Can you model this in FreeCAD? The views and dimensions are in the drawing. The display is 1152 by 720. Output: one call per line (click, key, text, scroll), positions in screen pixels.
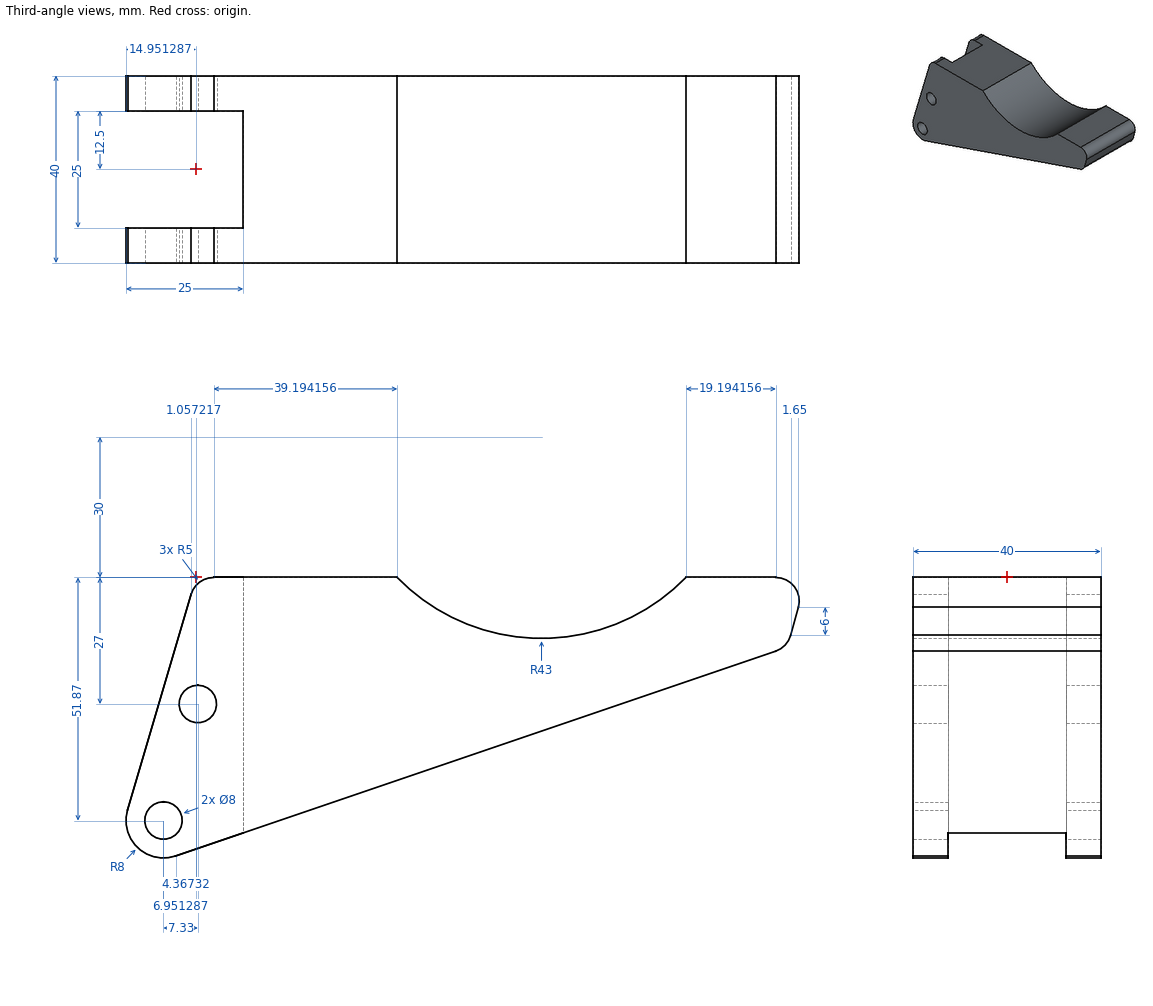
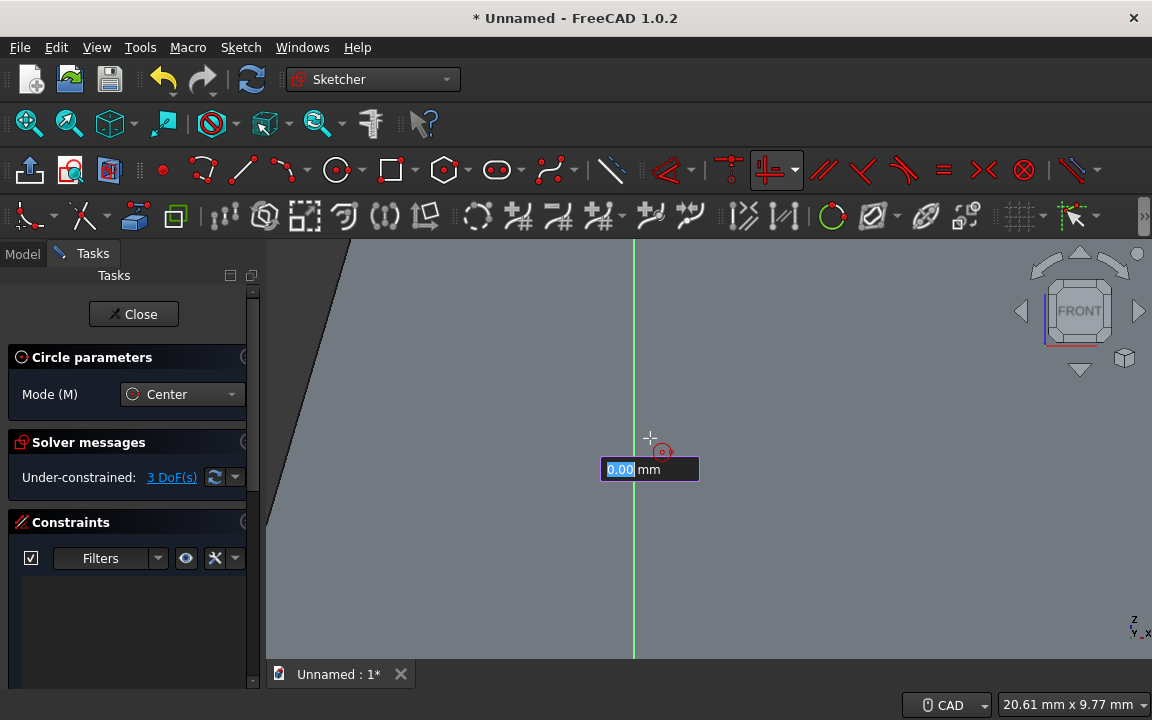
scroll(659, 445, down, 11)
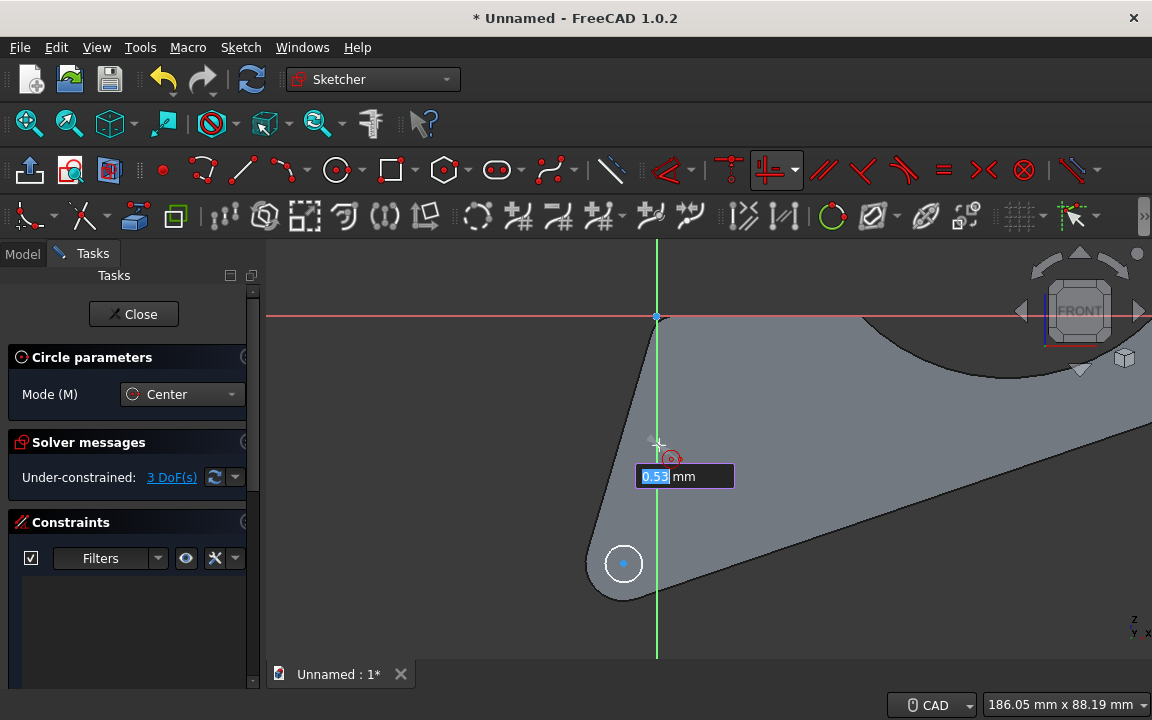
click(672, 431)
key(Escape)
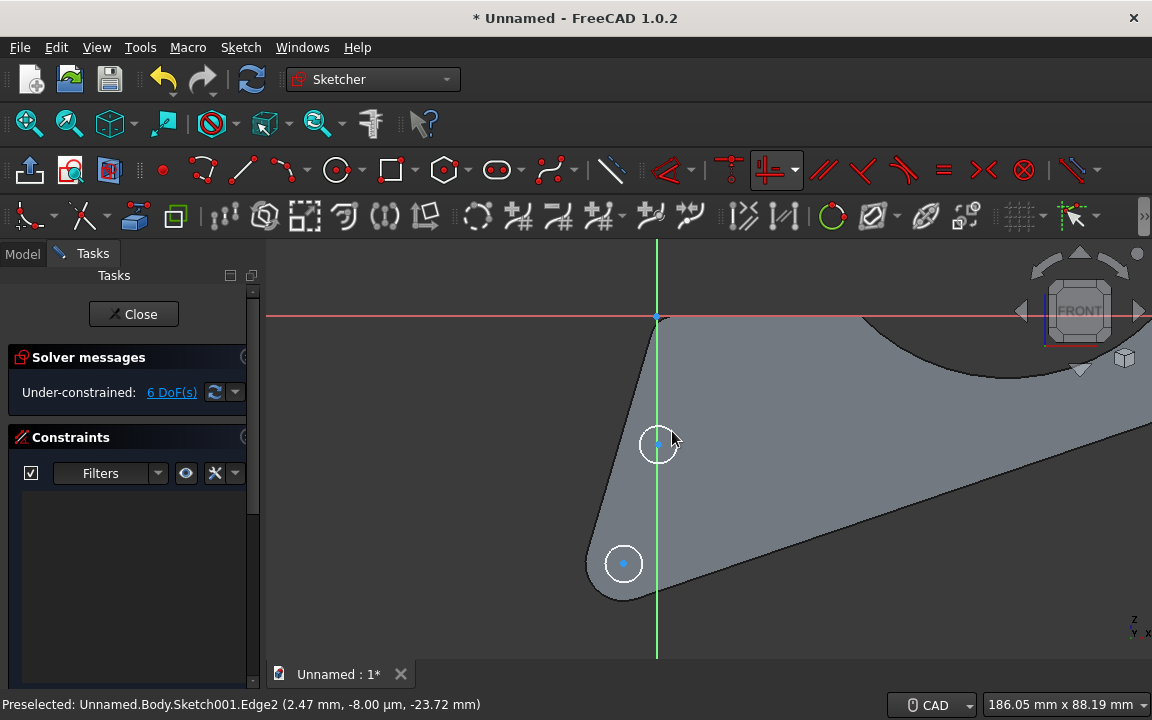
click(637, 551)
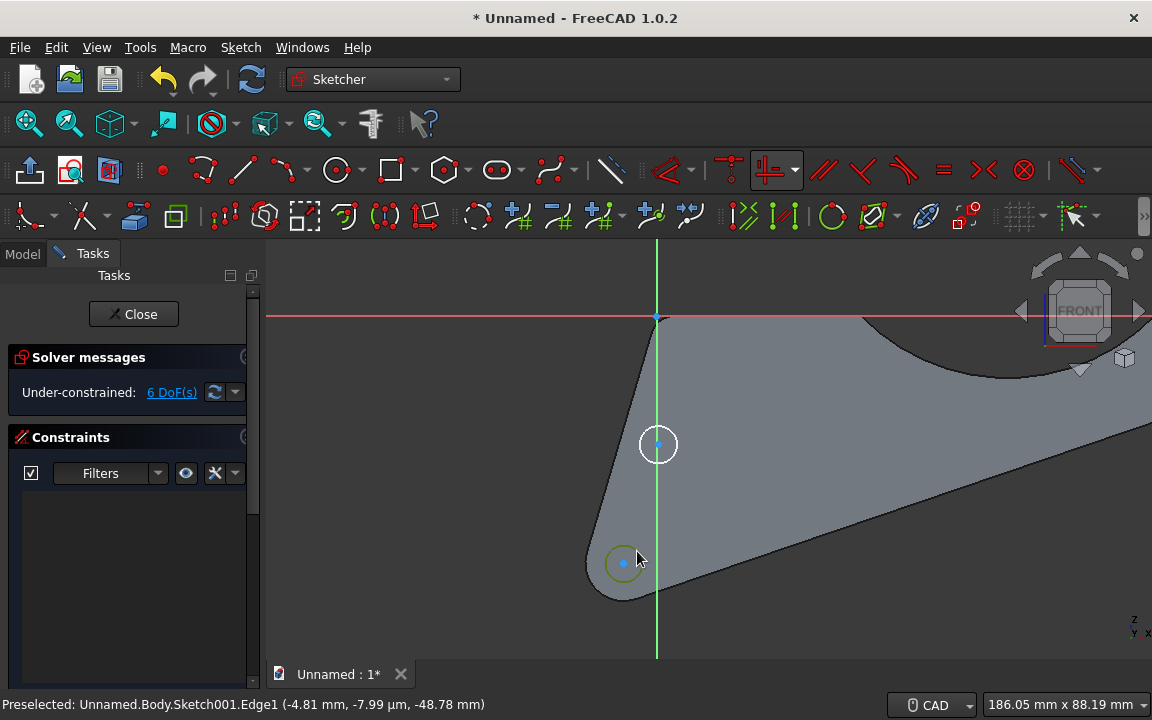
click(672, 432)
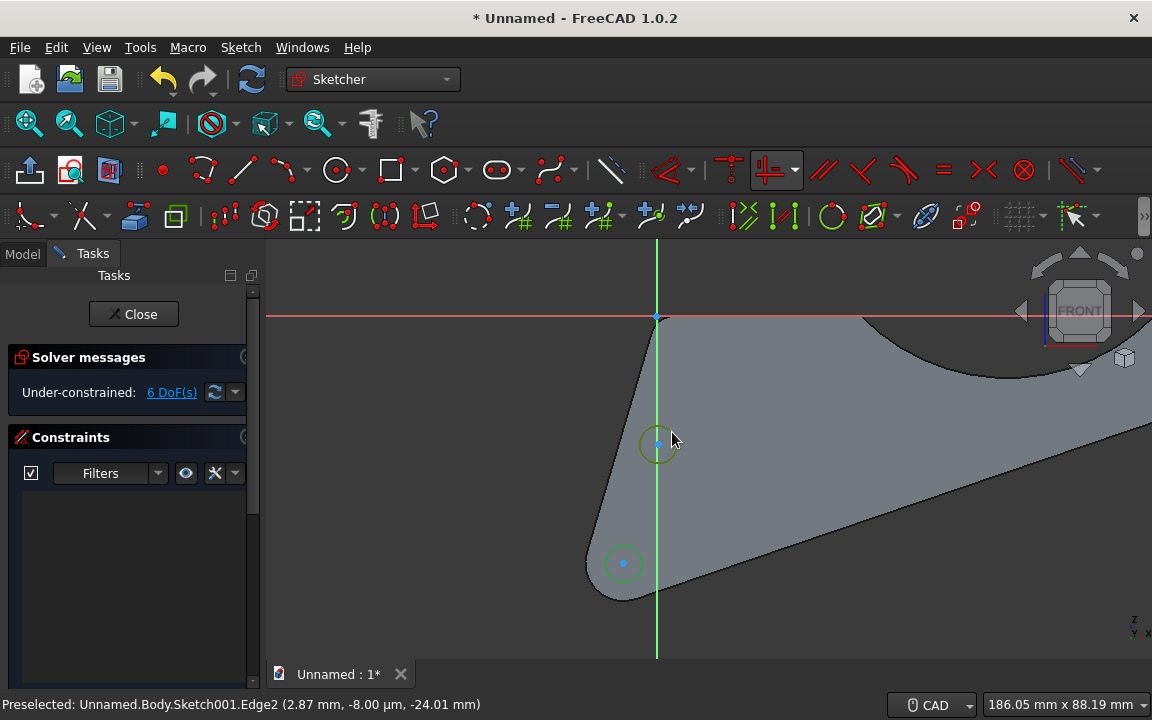
key(e)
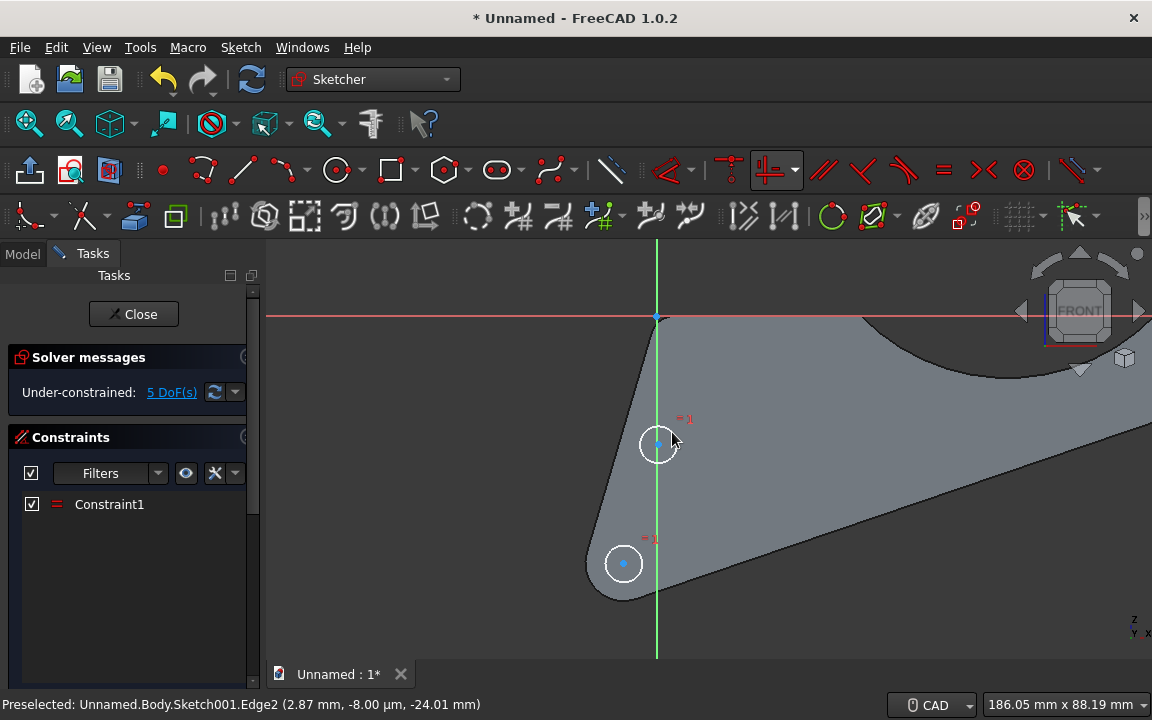
click(666, 170)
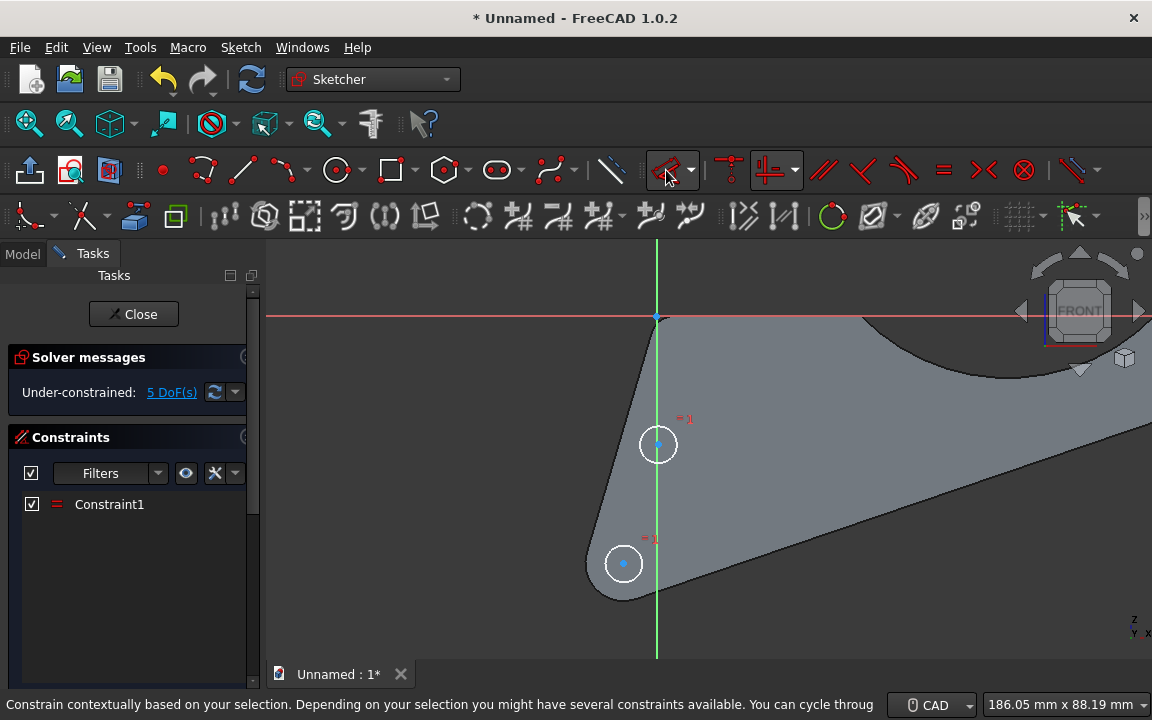
click(637, 551)
click(672, 550)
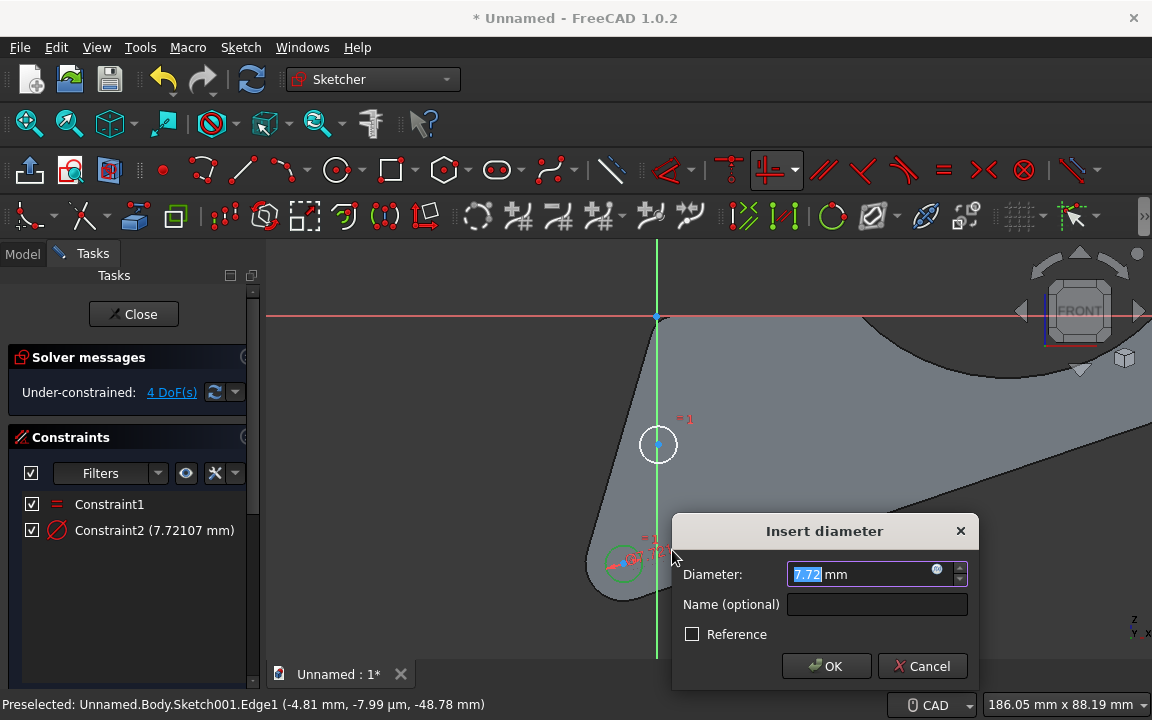
text(8)
key(Return)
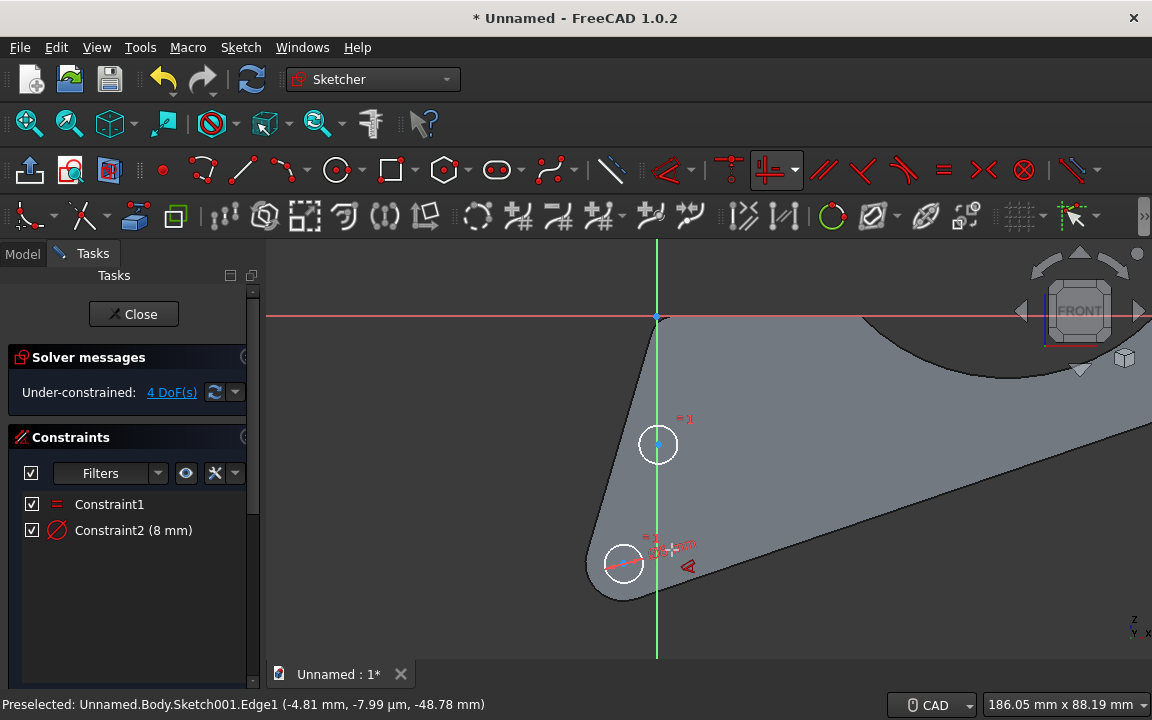
click(658, 445)
click(692, 380)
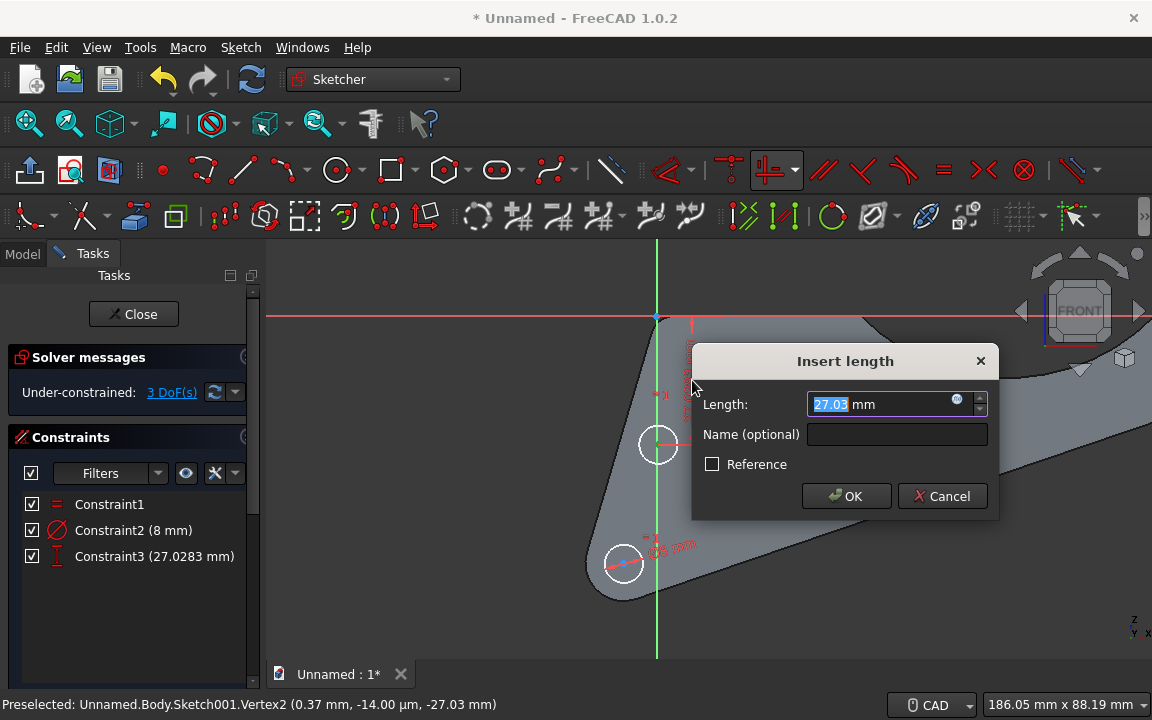
text(27)
key(Return)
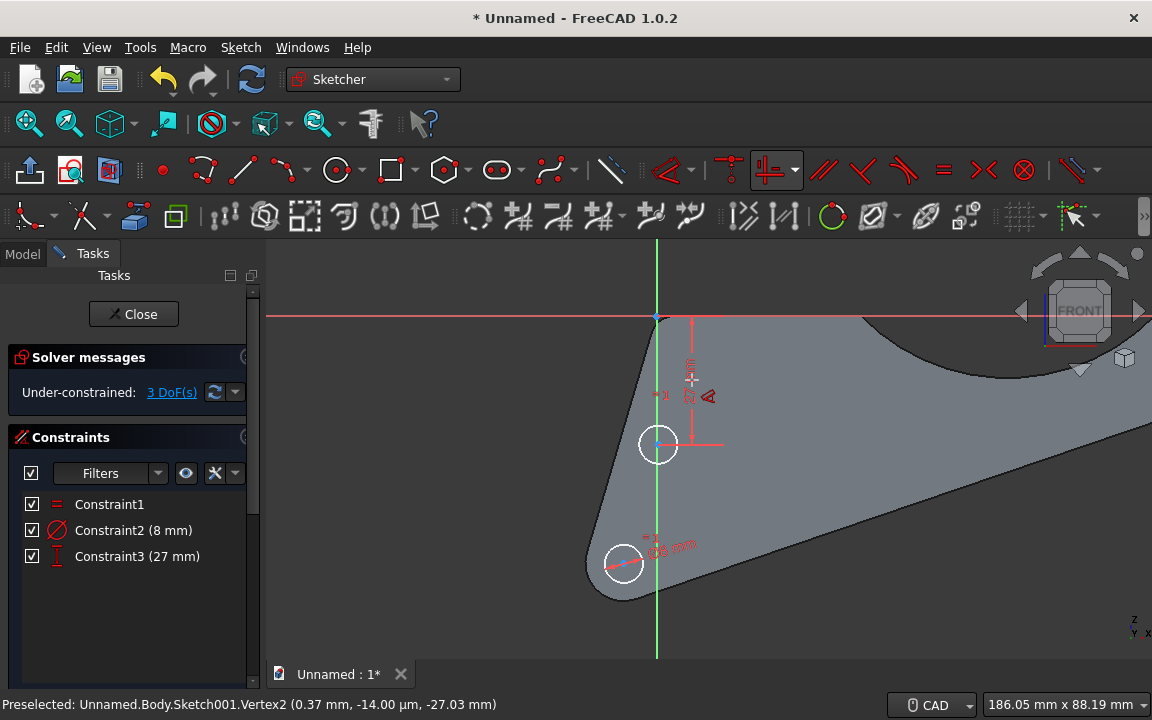
click(624, 564)
click(590, 440)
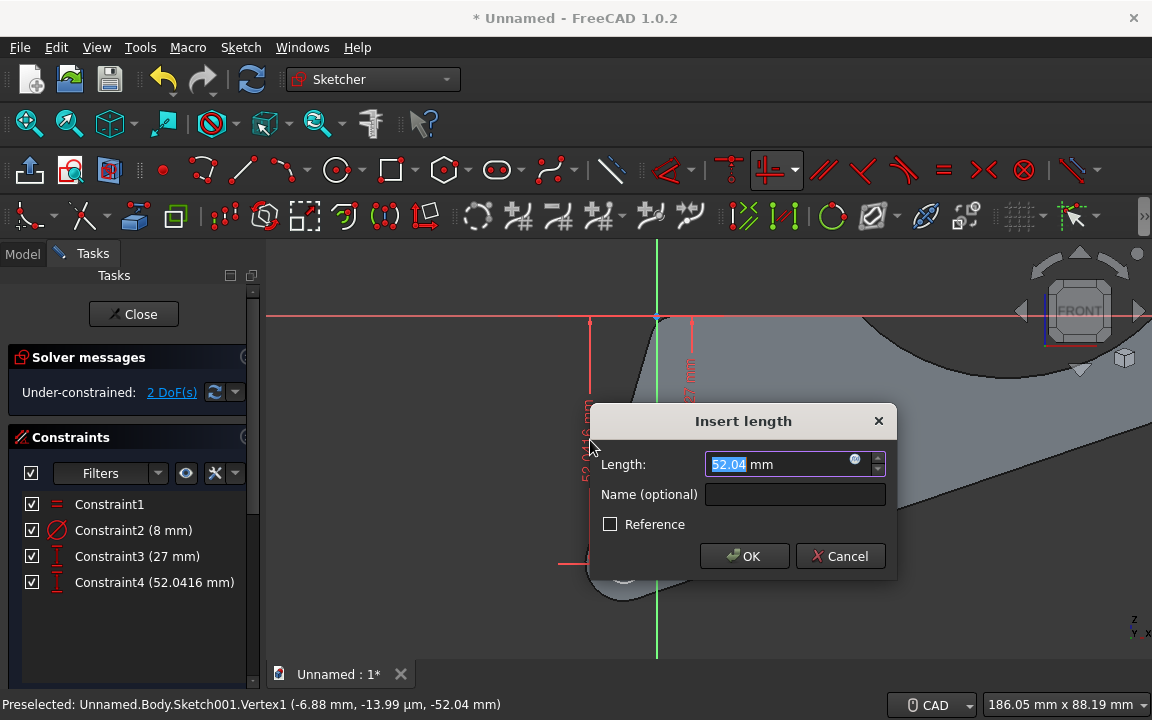
text(51.87)
key(Return)